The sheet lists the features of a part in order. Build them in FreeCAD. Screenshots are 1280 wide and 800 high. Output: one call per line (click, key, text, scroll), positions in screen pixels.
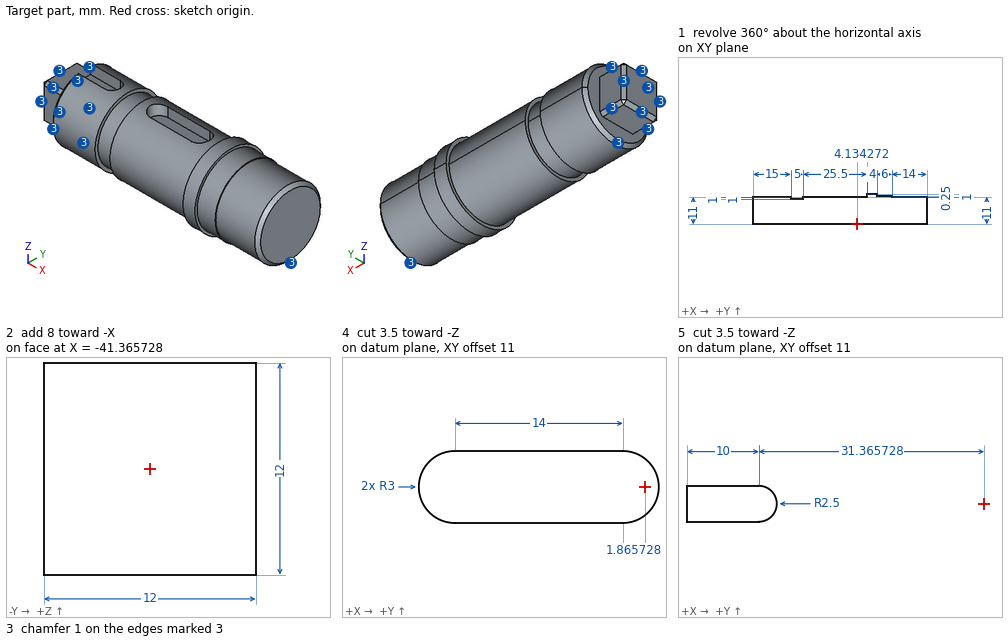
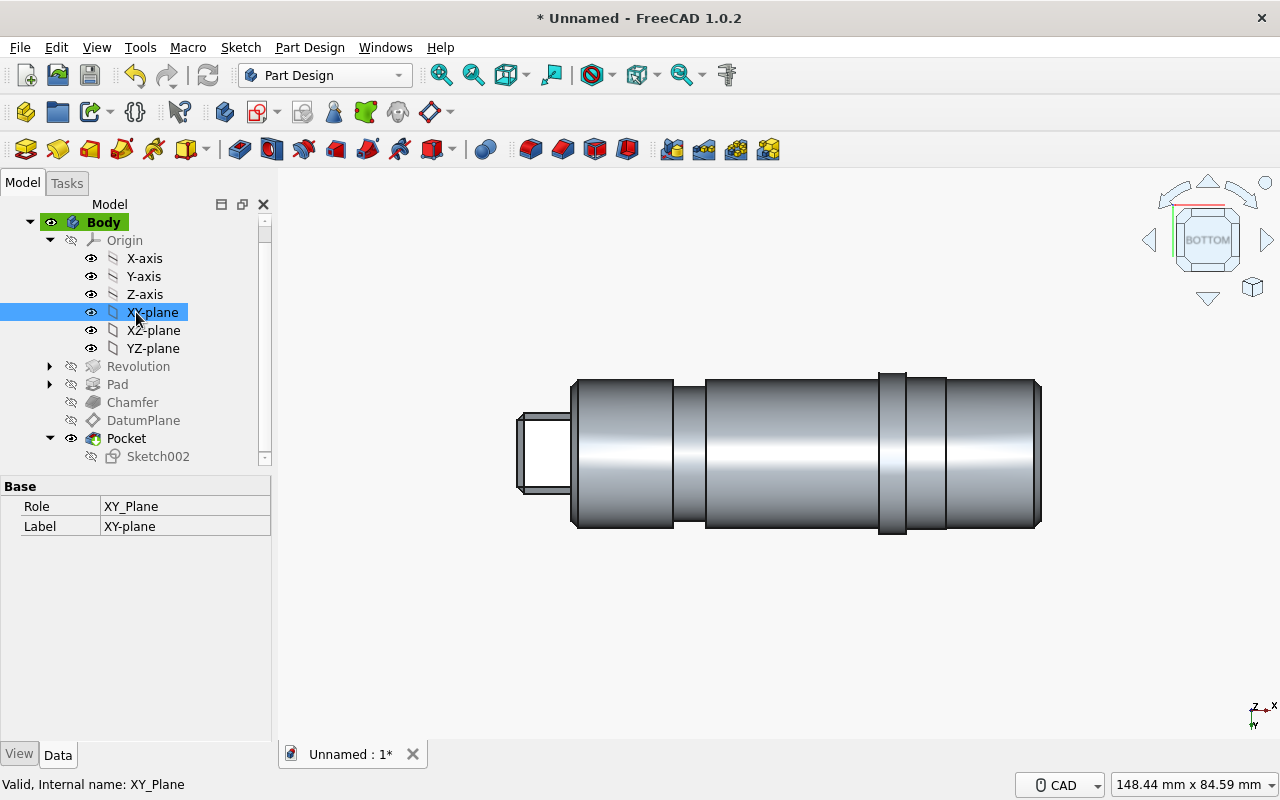
click(430, 112)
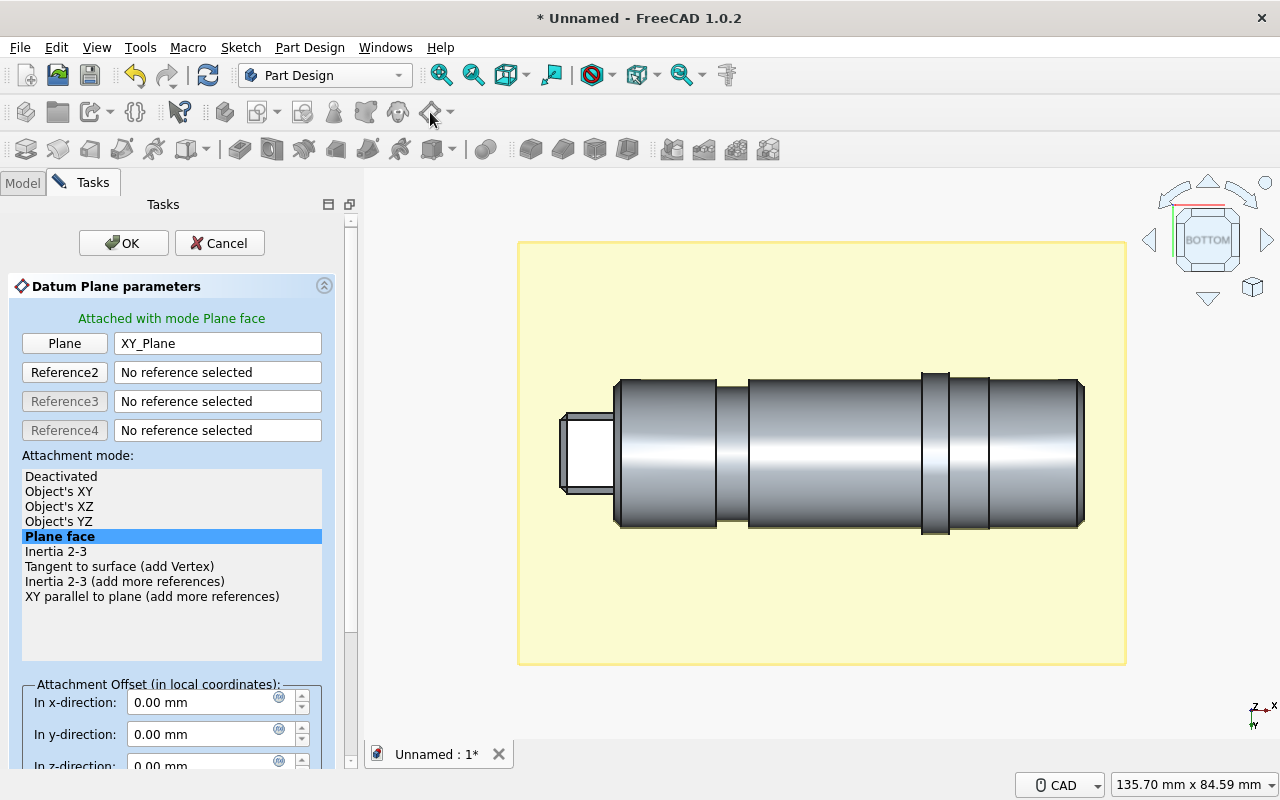
scroll(351, 491, down, 2)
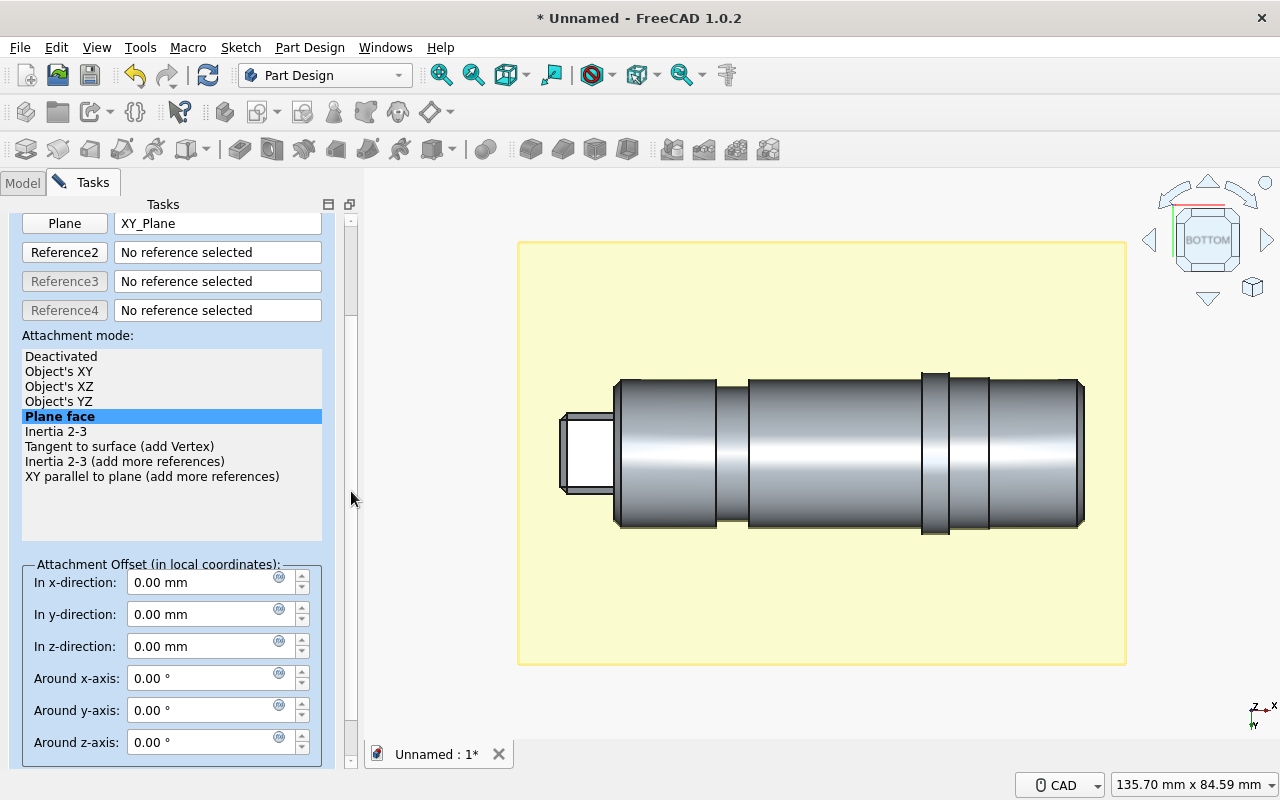
triple_click(210, 646)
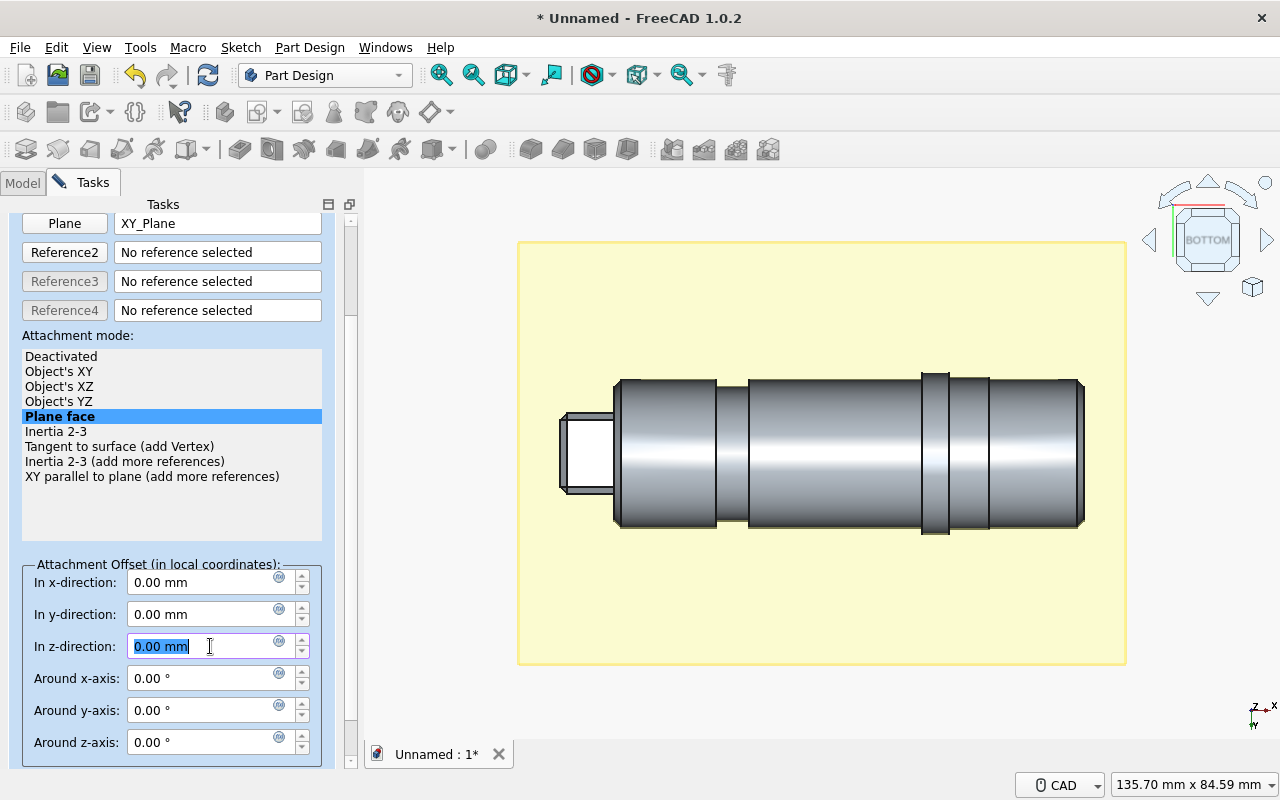
text(11)
key(Tab)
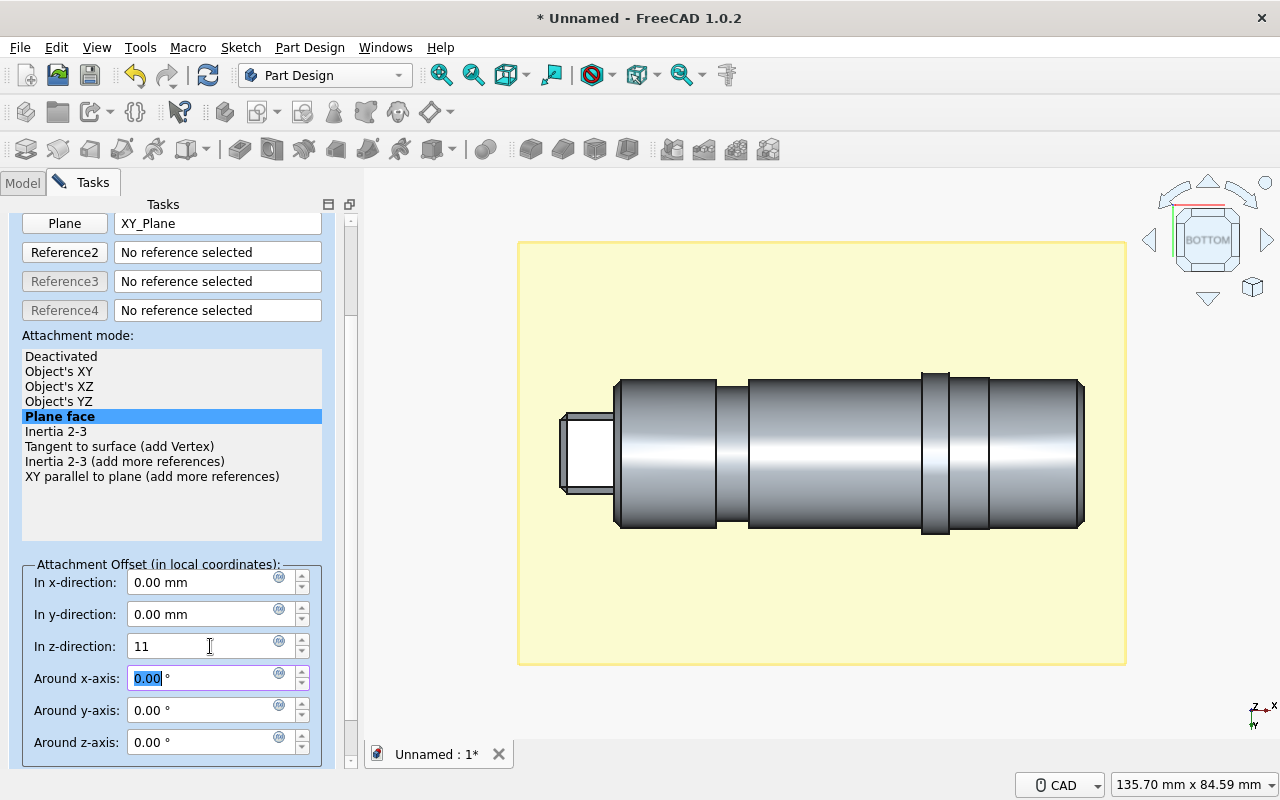
scroll(351, 491, up, 3)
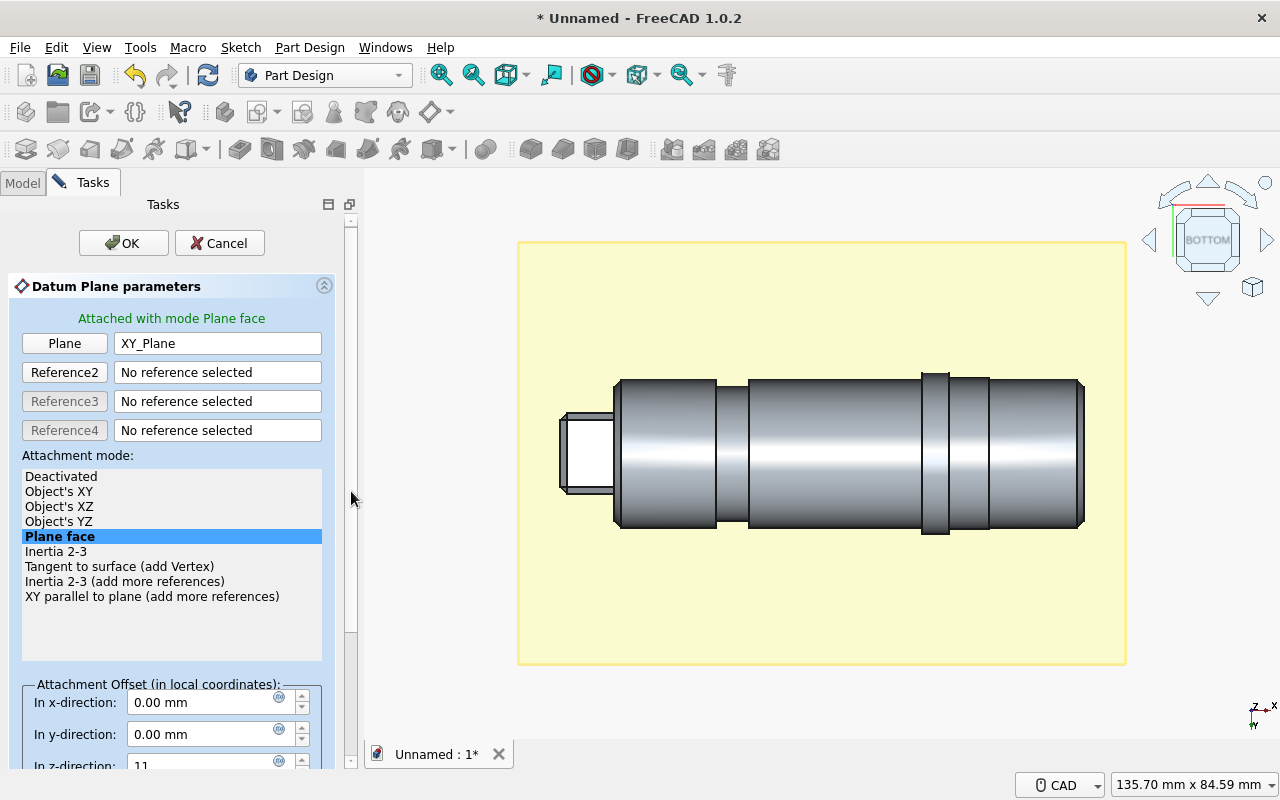
click(124, 243)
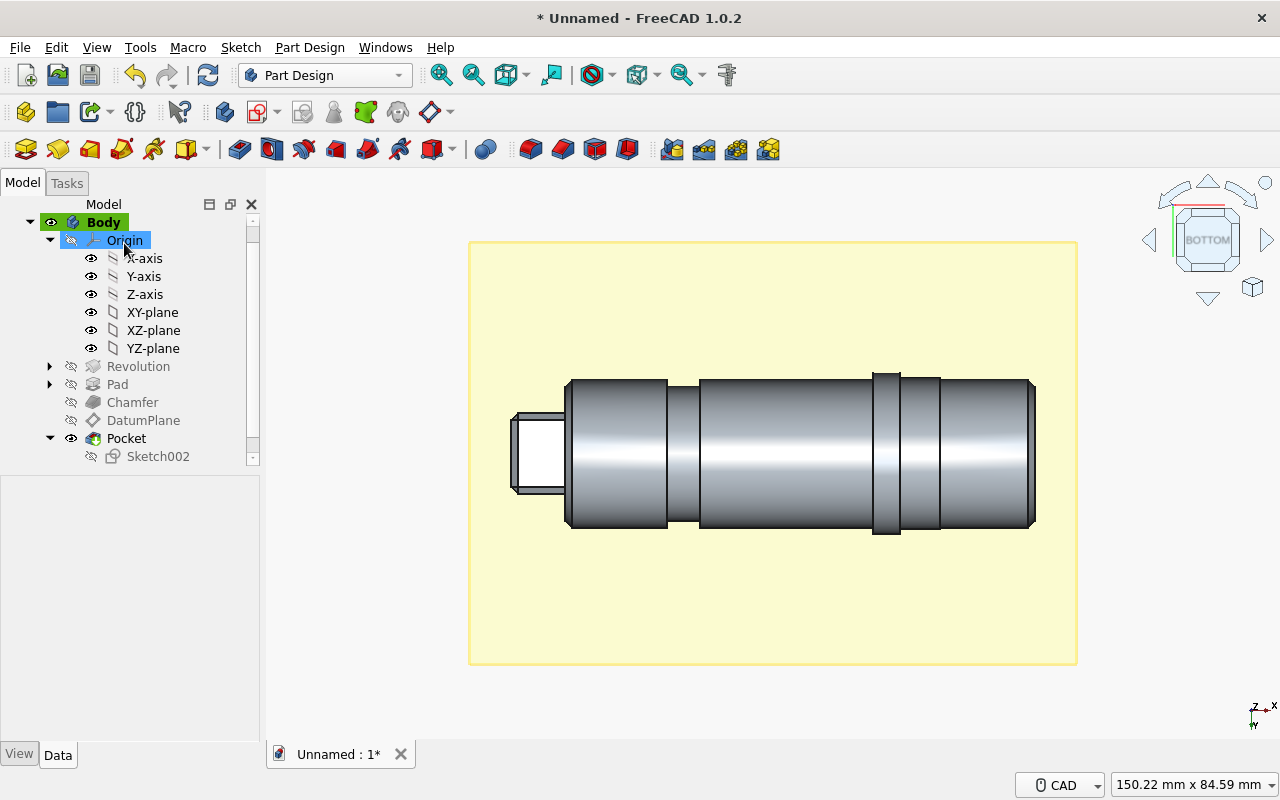
scroll(120, 344, down, 3)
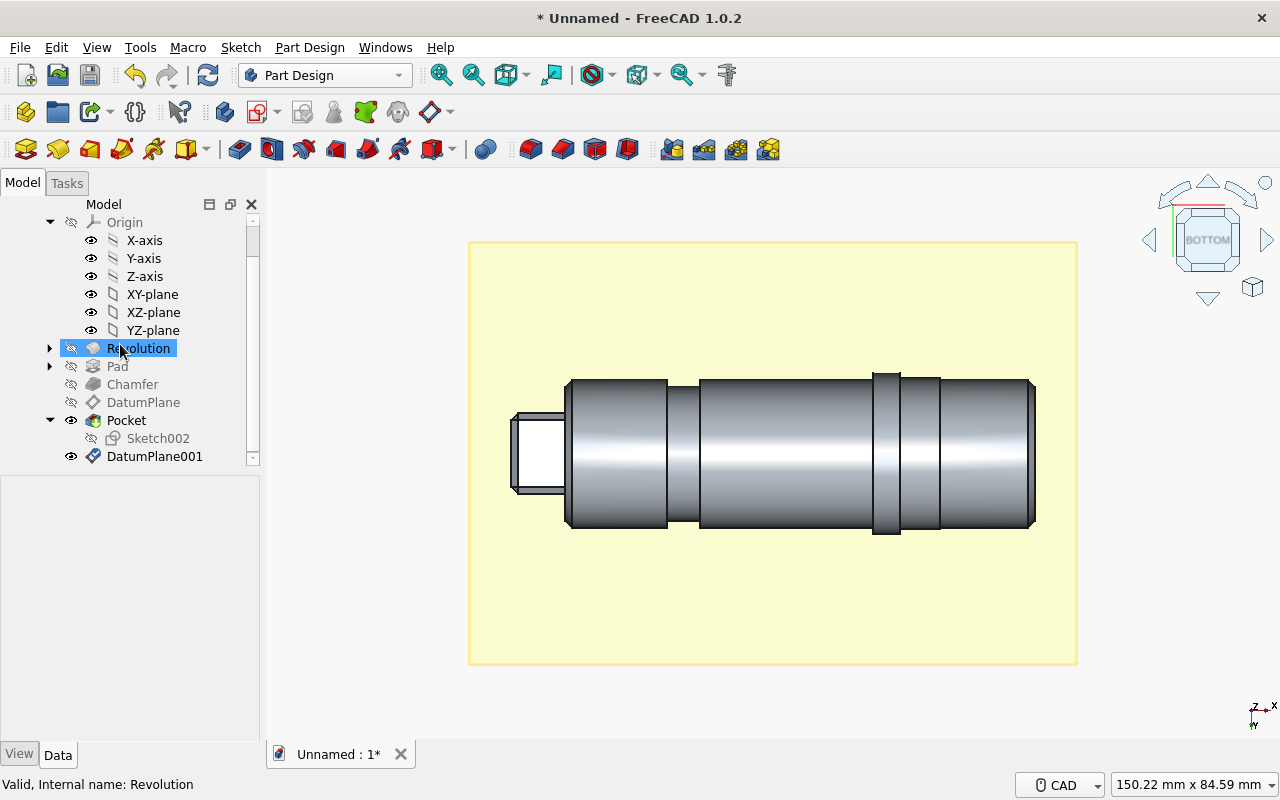
click(116, 456)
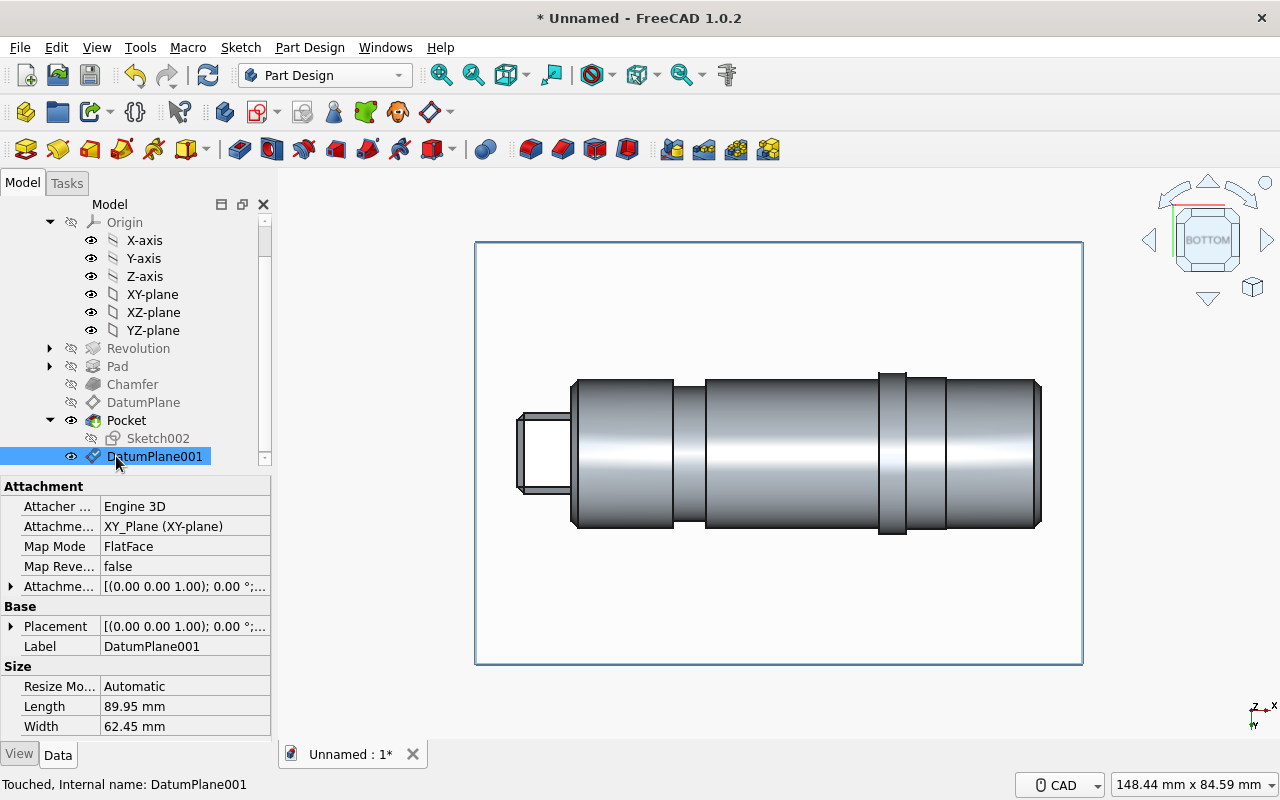
click(258, 112)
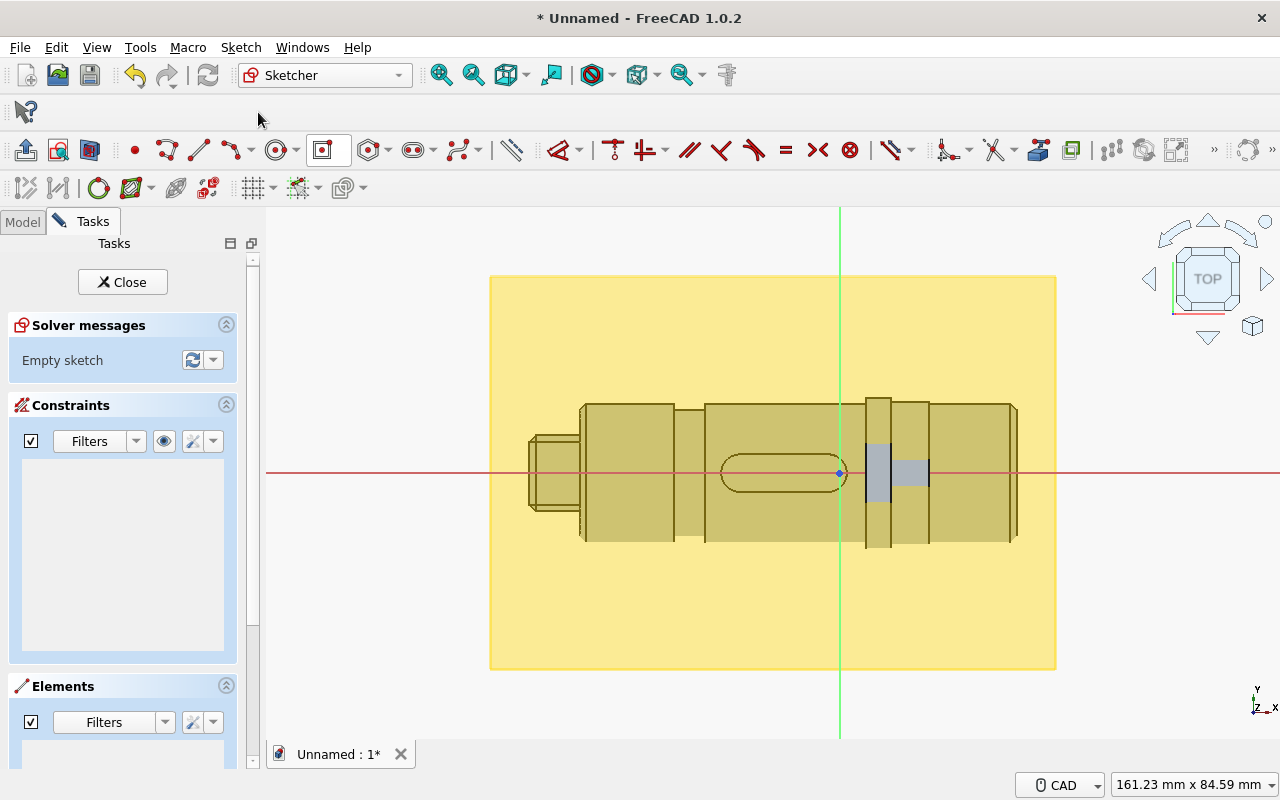
key(q)
key(s)